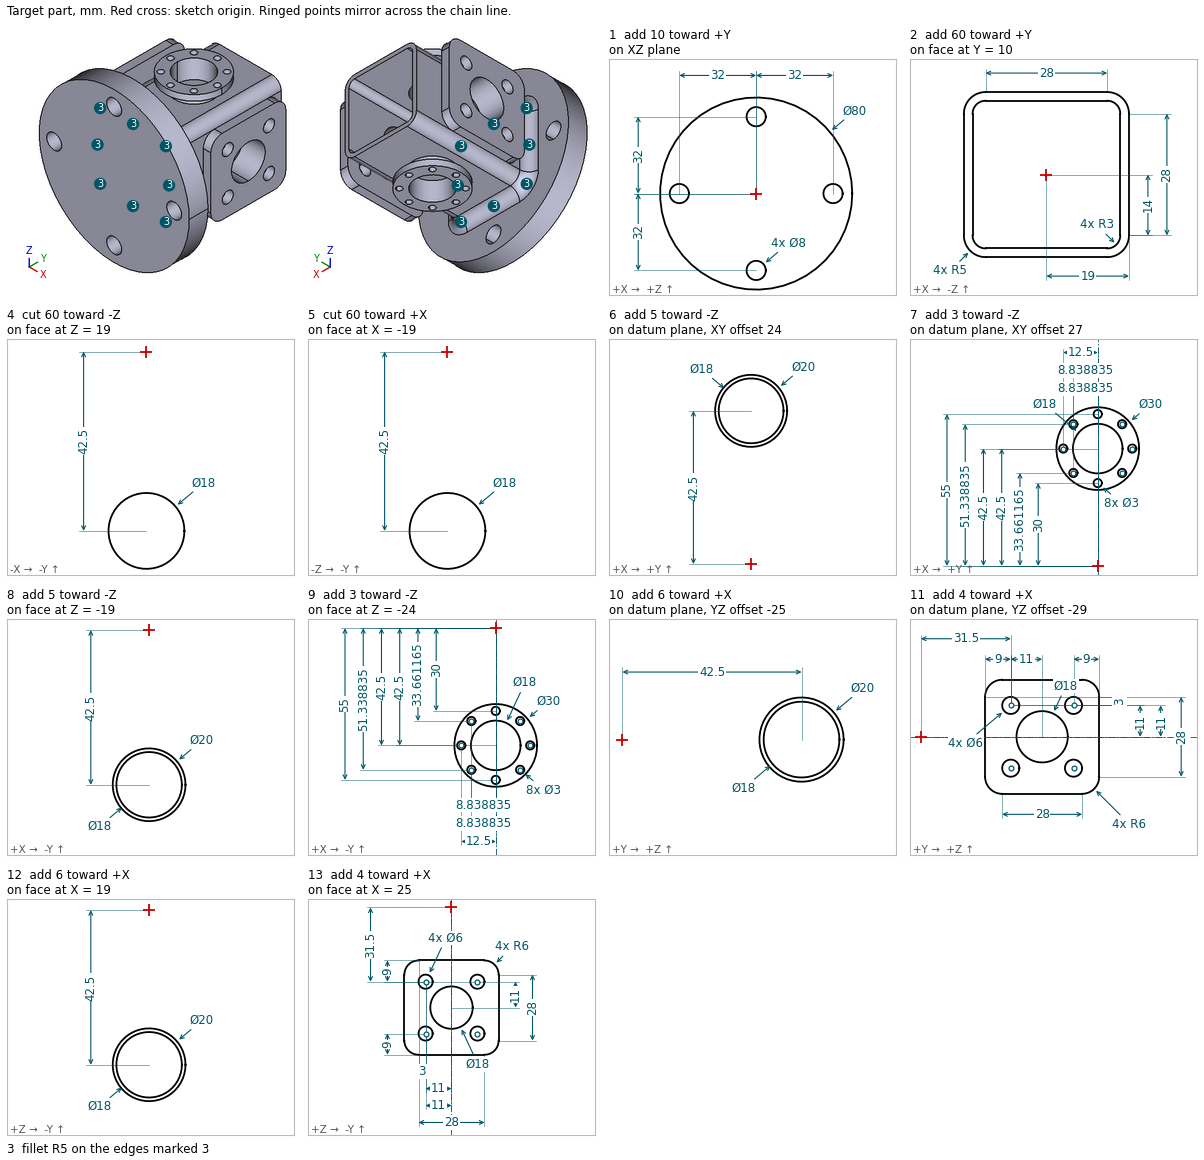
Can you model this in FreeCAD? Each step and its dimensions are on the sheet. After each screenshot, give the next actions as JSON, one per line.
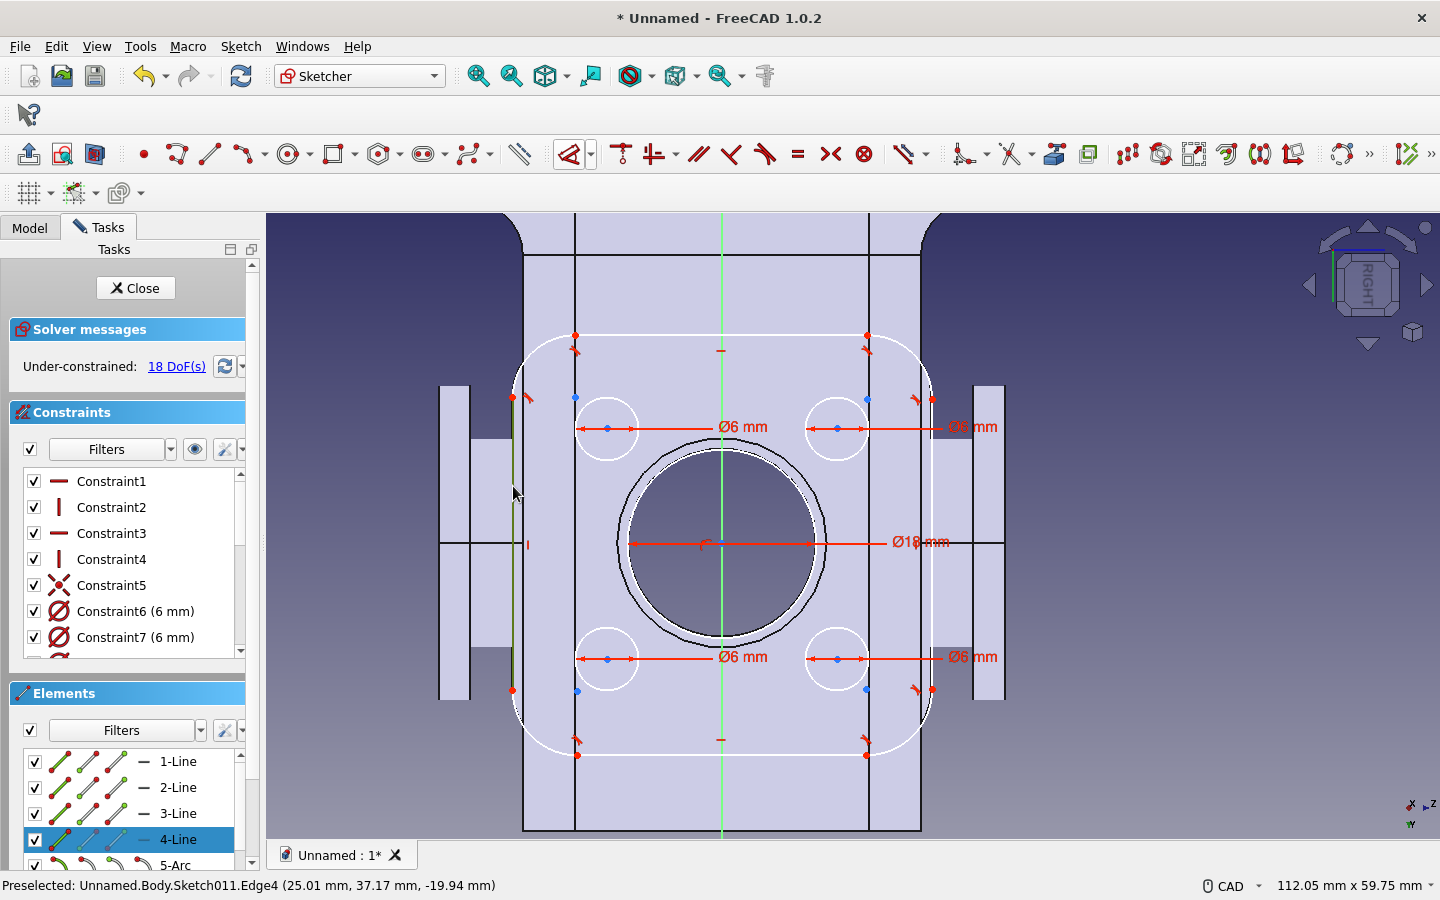
{"action": "left_click", "coordinate": [520, 720]}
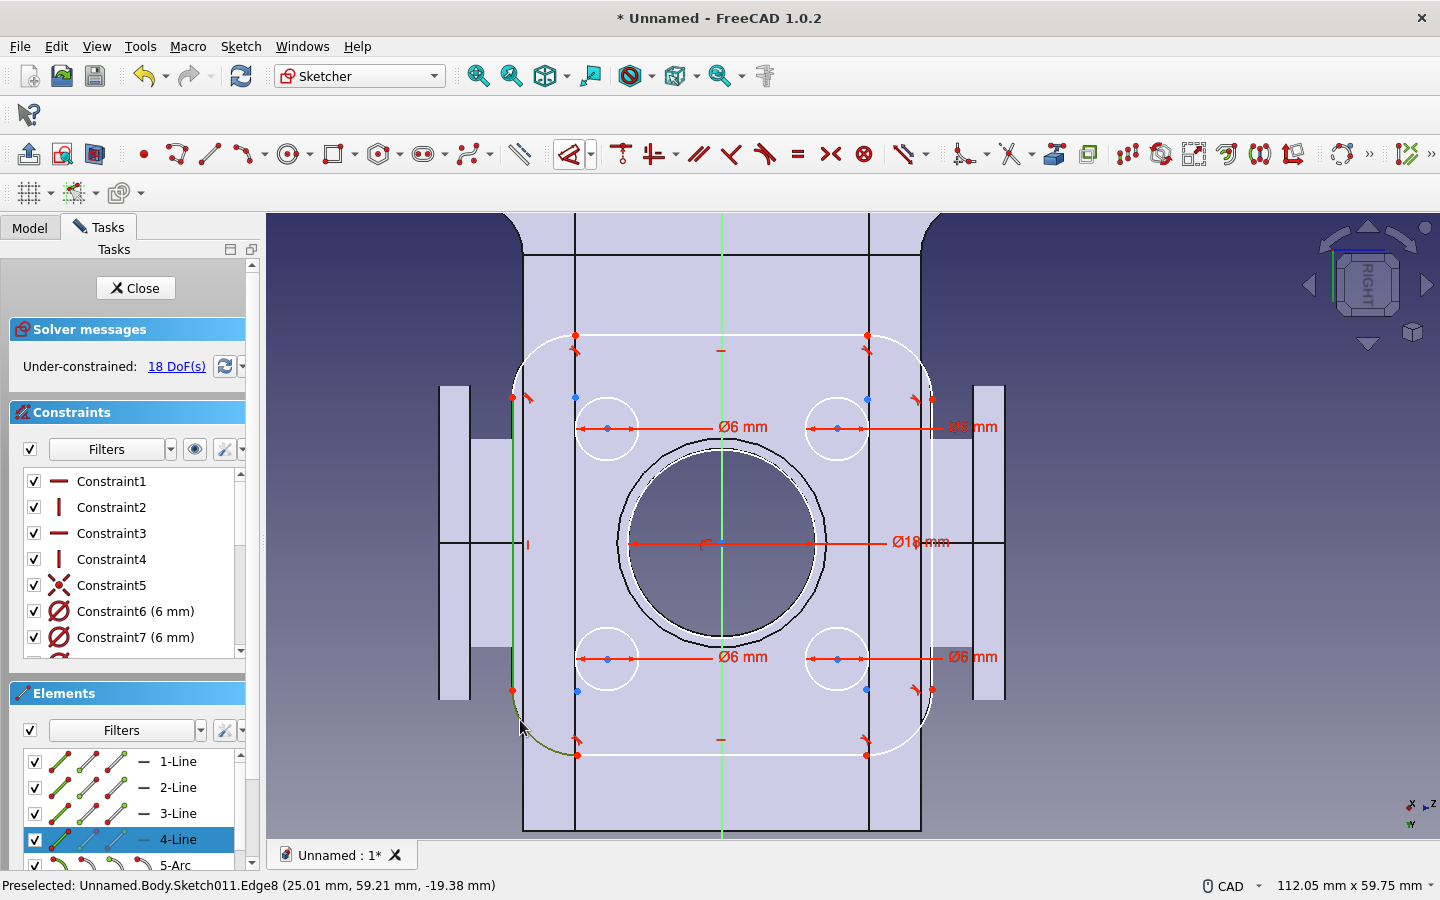
{"action": "key", "text": "t"}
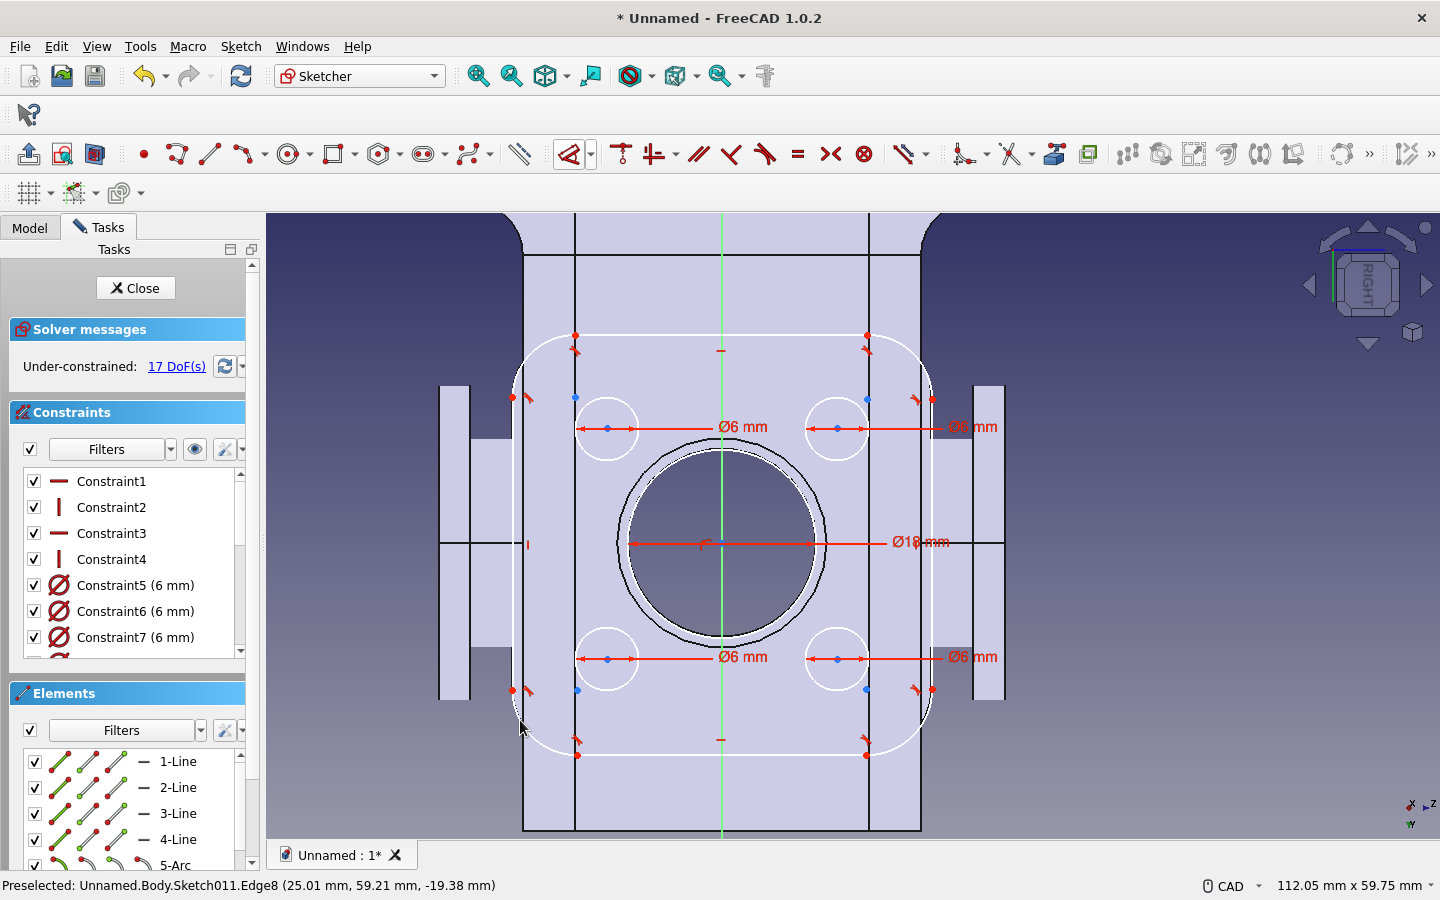
{"action": "left_click", "coordinate": [896, 748]}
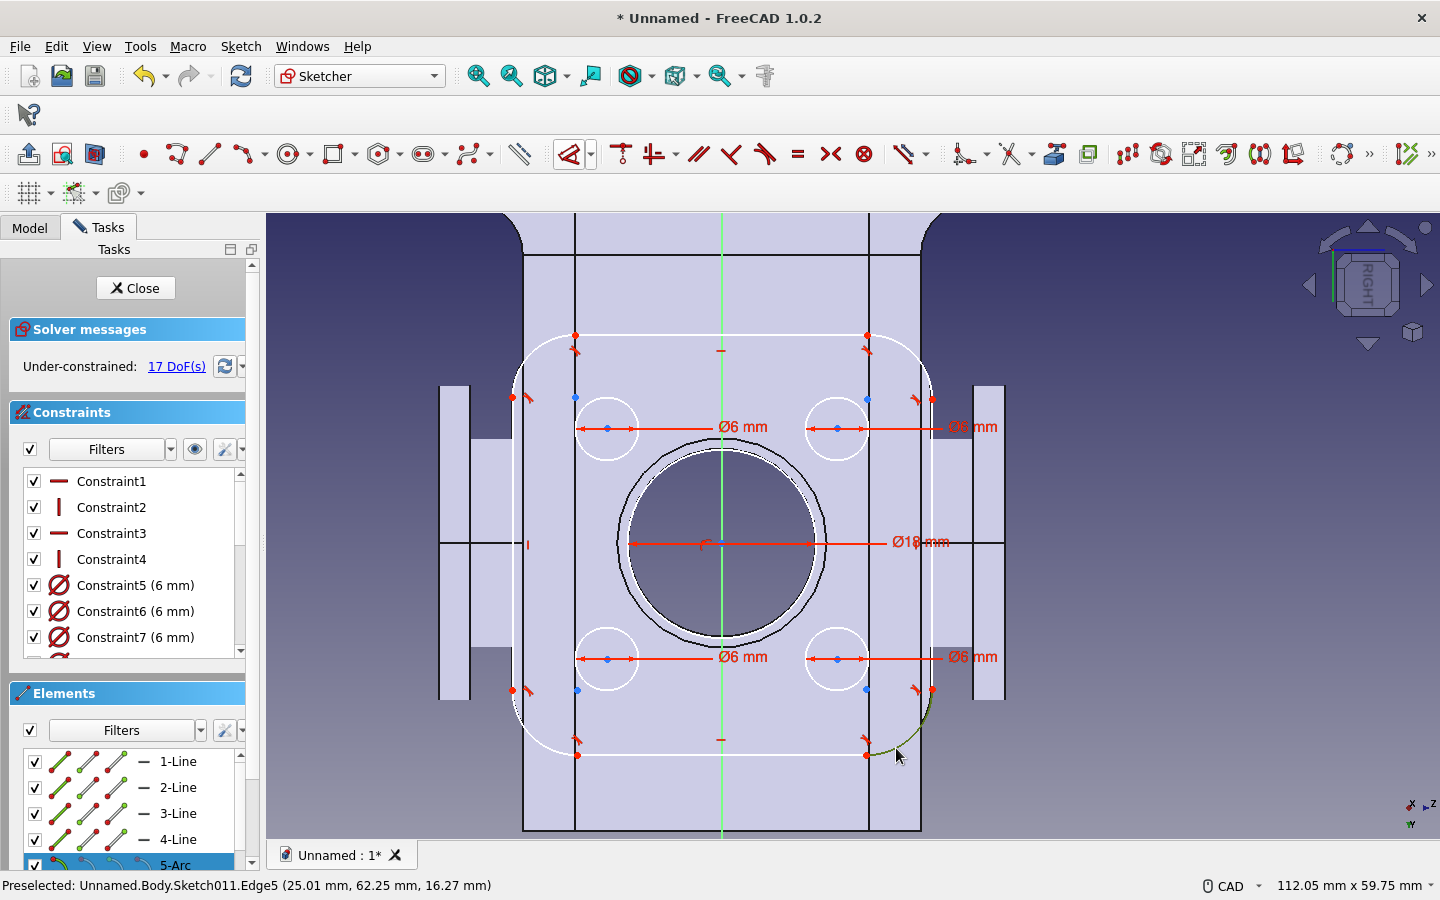
{"action": "left_click", "coordinate": [925, 370]}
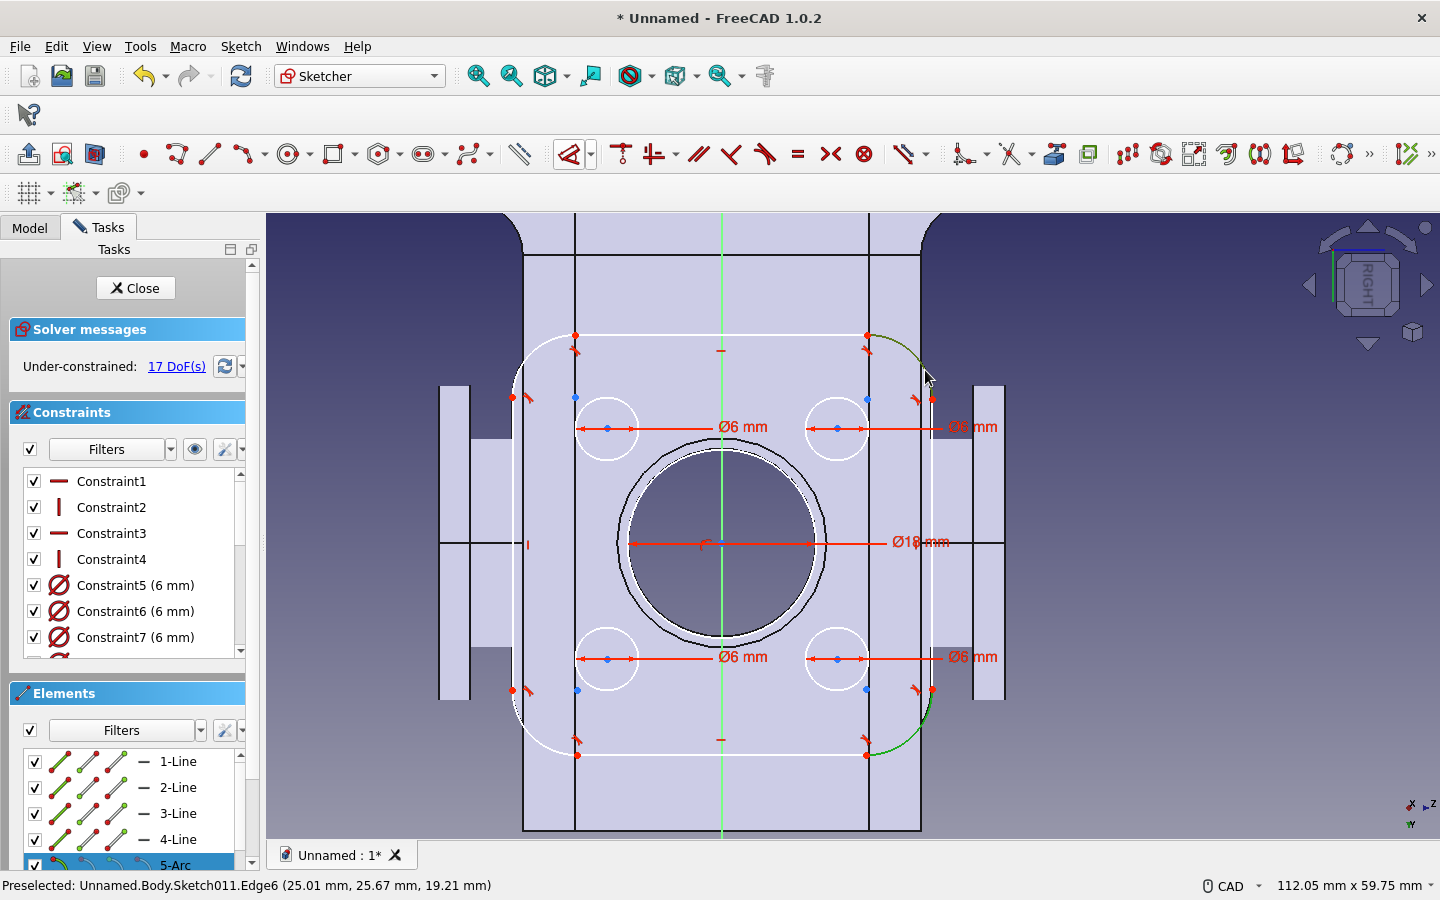
{"action": "left_click", "coordinate": [547, 342]}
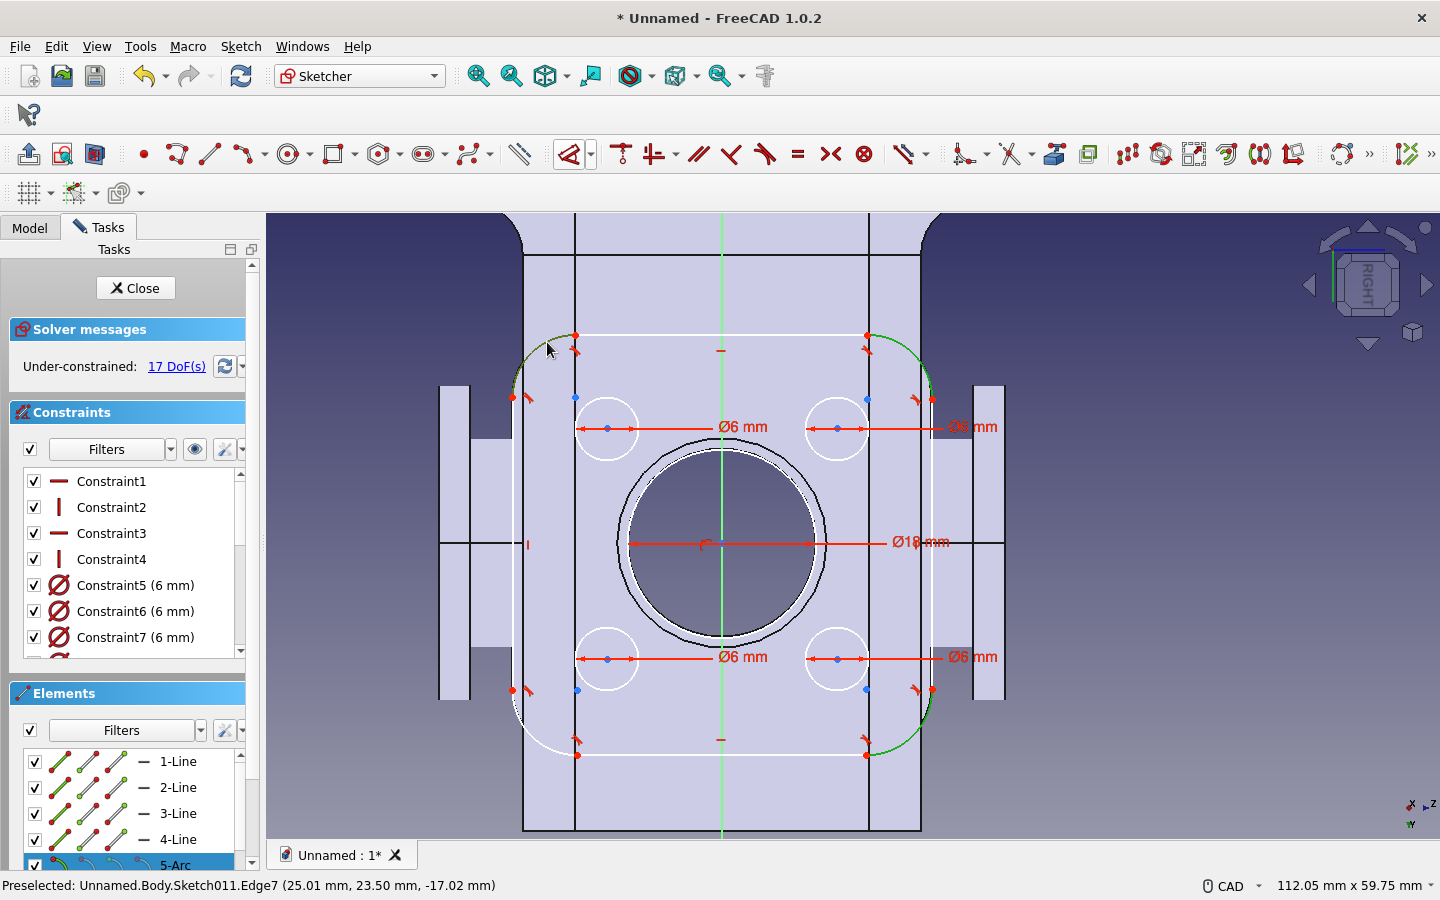
{"action": "left_click", "coordinate": [520, 720]}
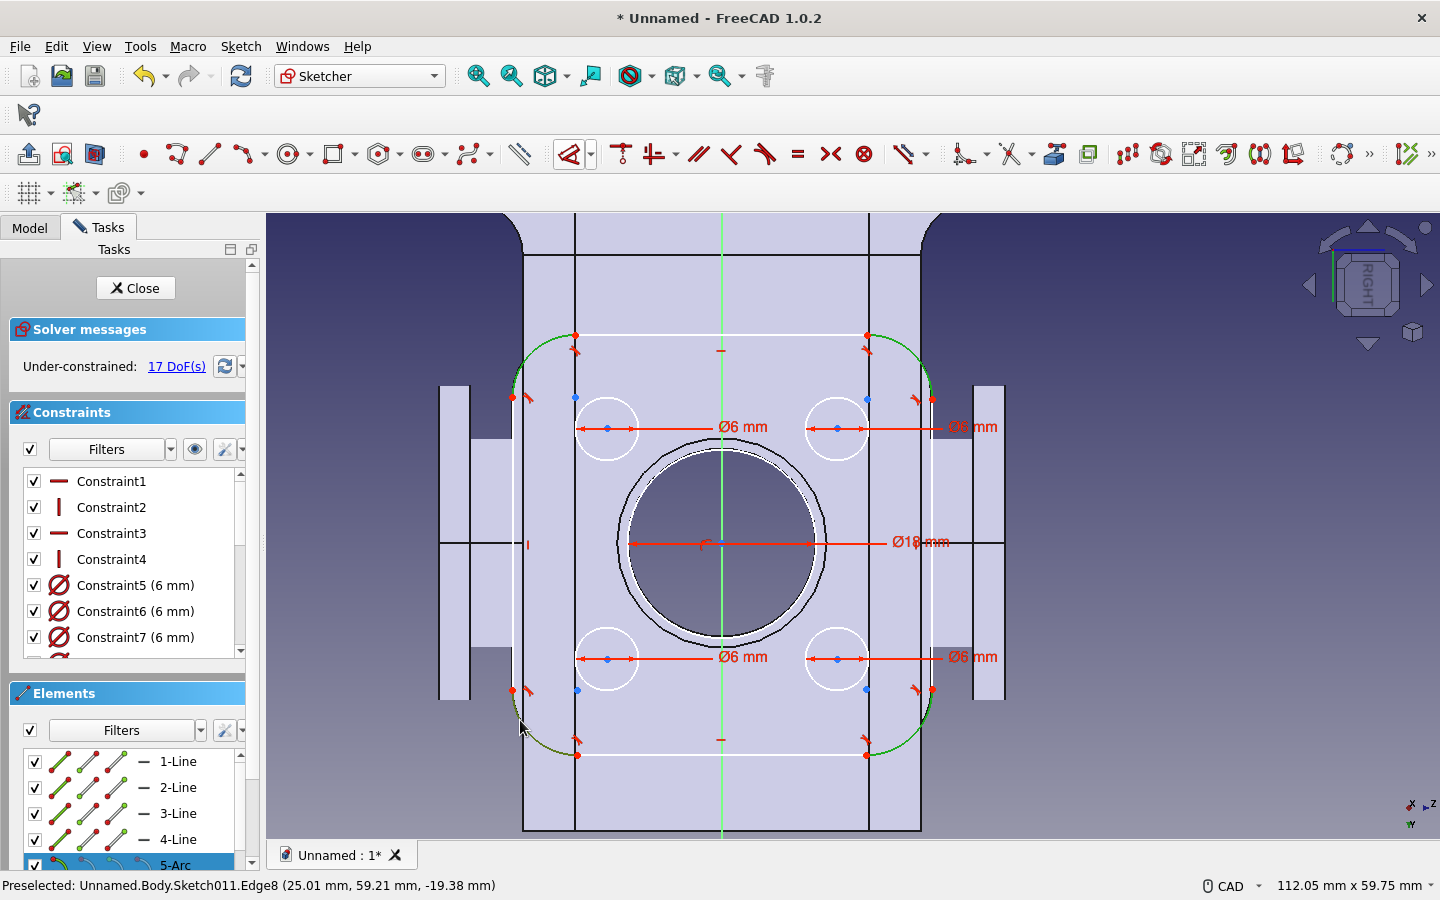
{"action": "key", "text": "e"}